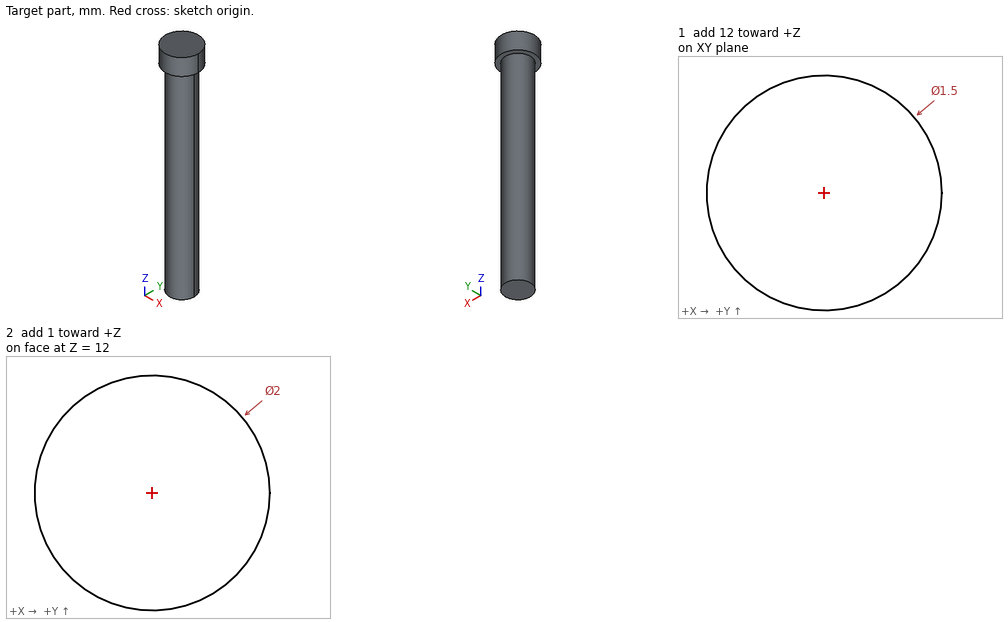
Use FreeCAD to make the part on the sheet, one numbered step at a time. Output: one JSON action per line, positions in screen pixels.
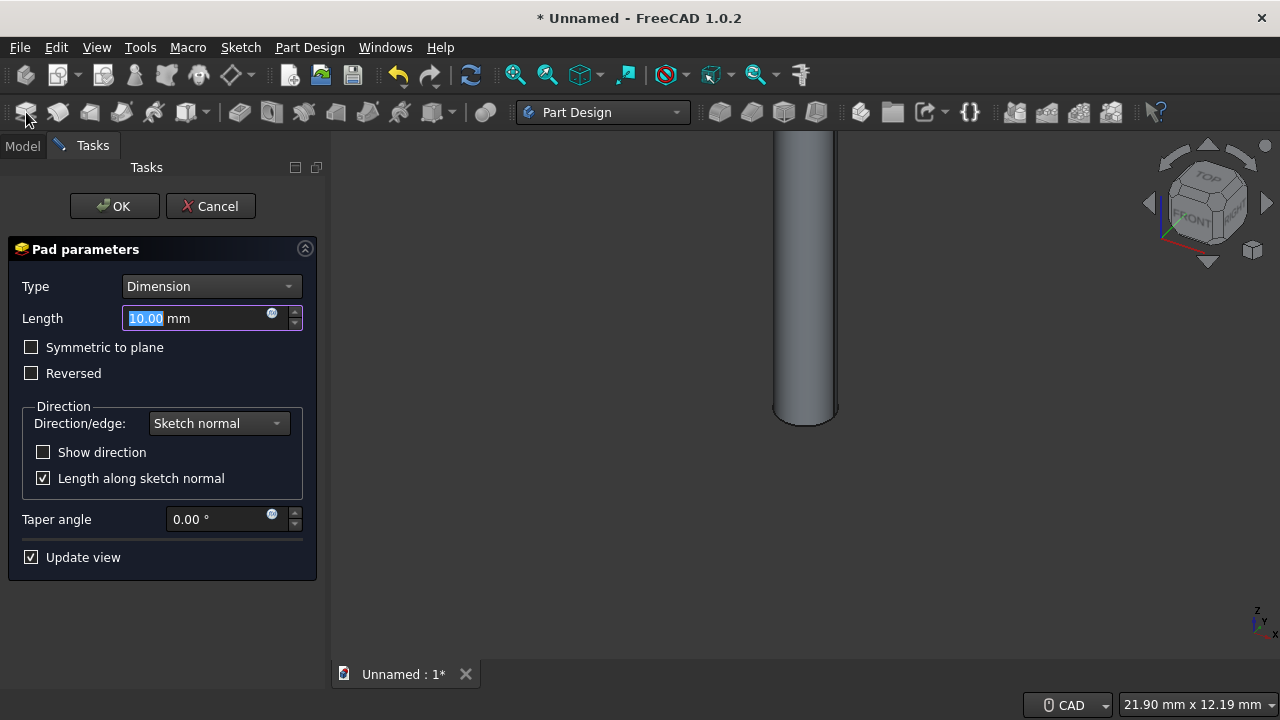
{"action": "type", "text": "1"}
{"action": "key", "text": "Tab"}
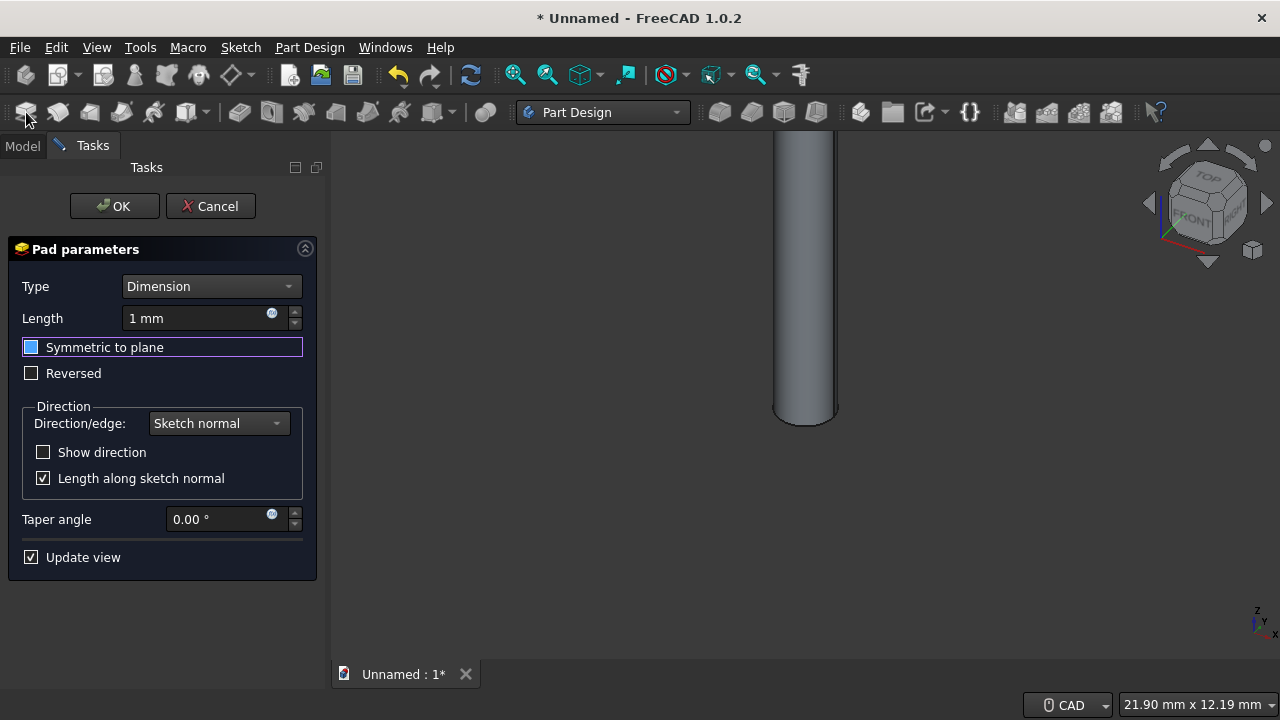
{"action": "left_click", "coordinate": [115, 206]}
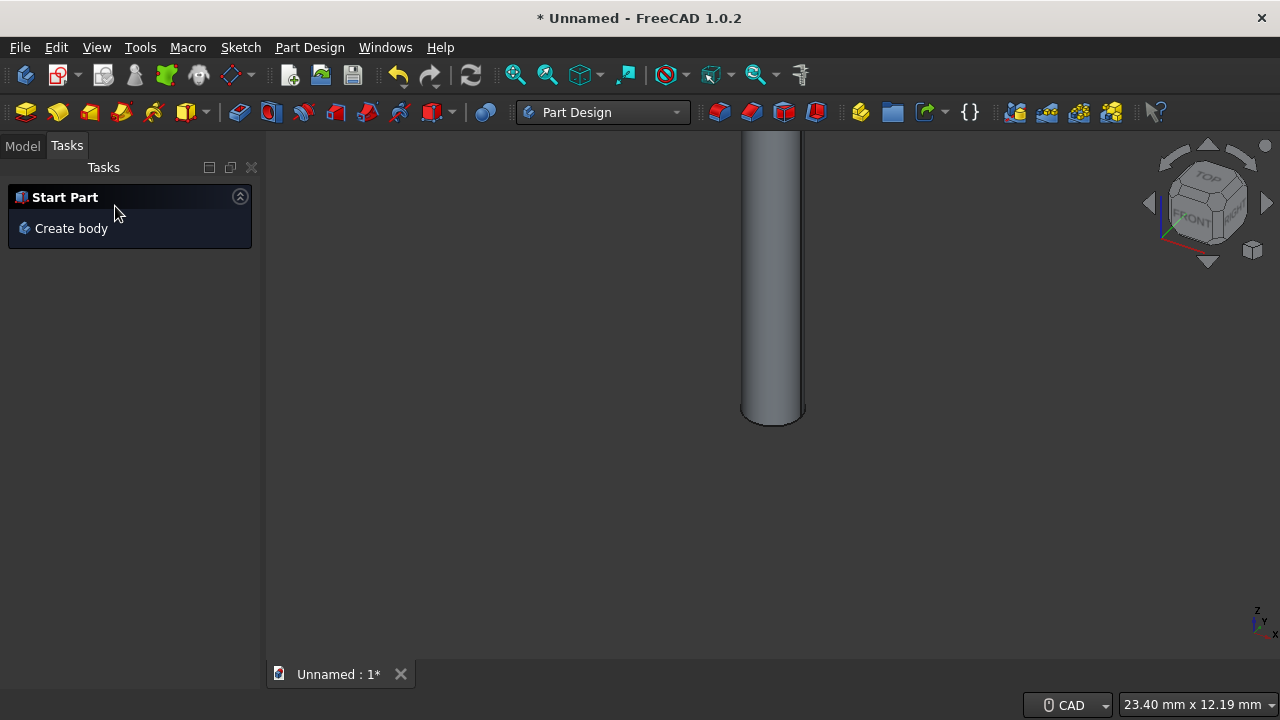
{"action": "key", "text": "0"}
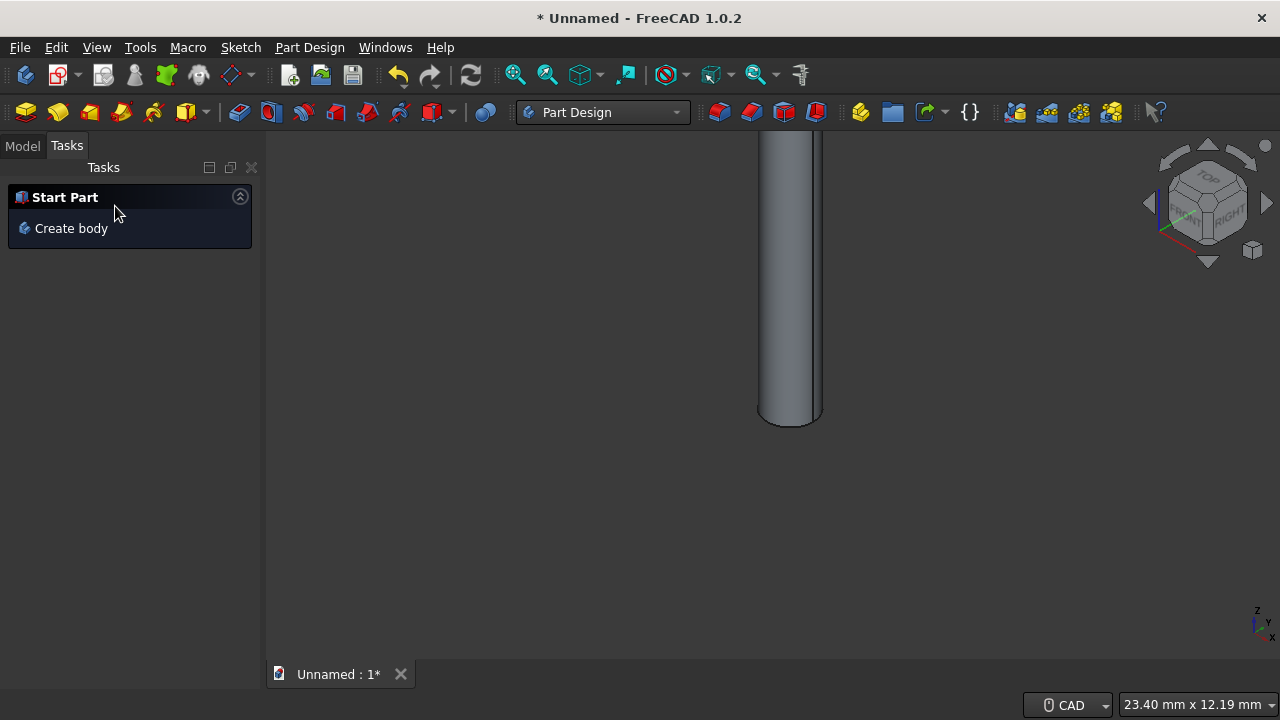
{"action": "left_click", "coordinate": [516, 76]}